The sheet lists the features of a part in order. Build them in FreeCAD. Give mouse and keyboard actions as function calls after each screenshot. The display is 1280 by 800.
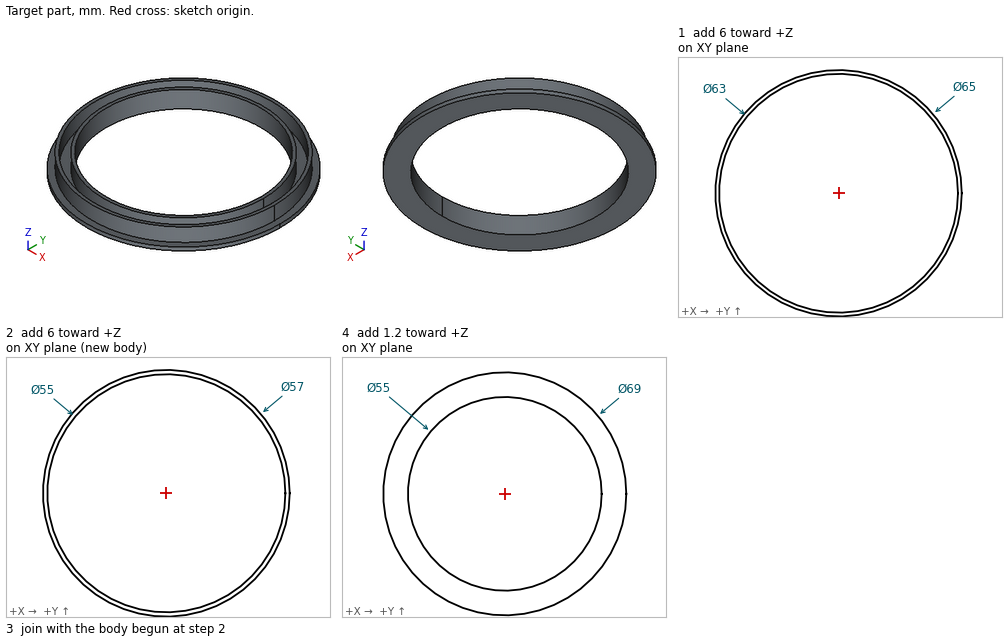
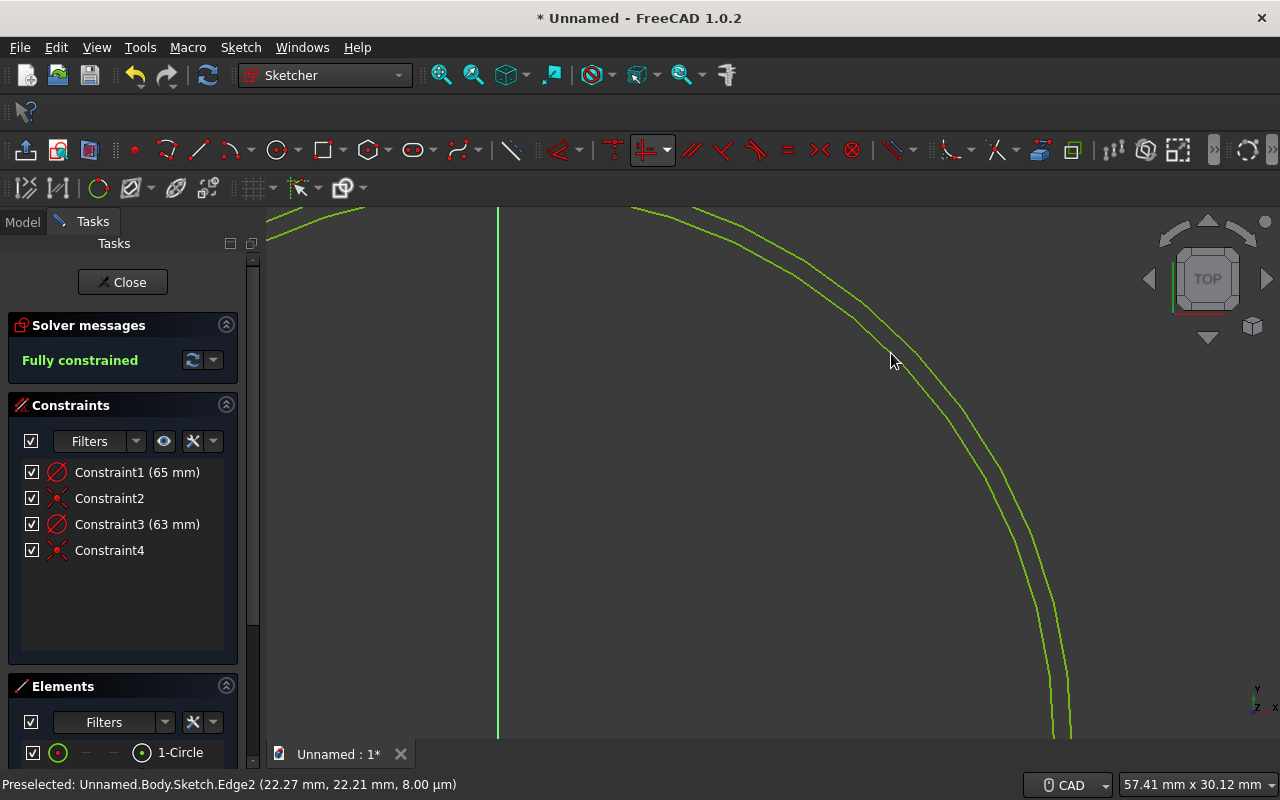
click(123, 282)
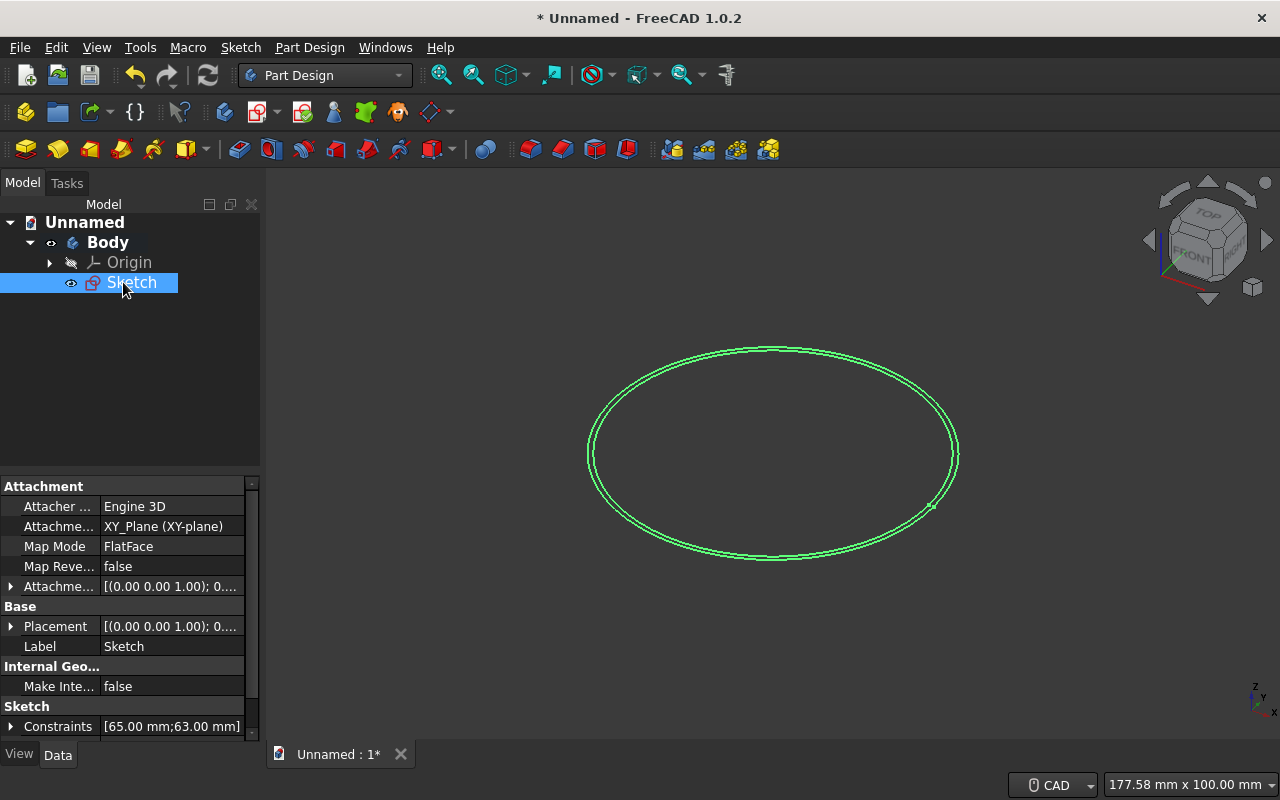
click(26, 150)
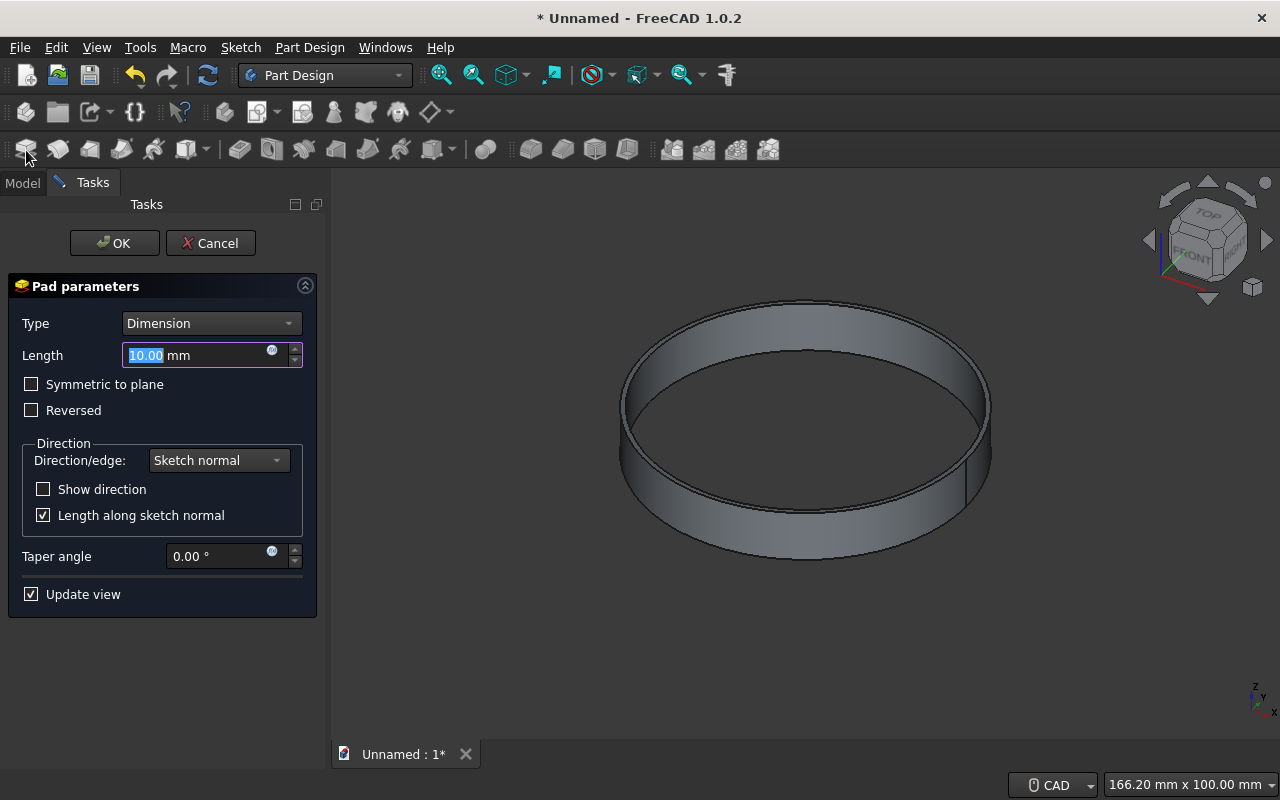
text(6)
key(Tab)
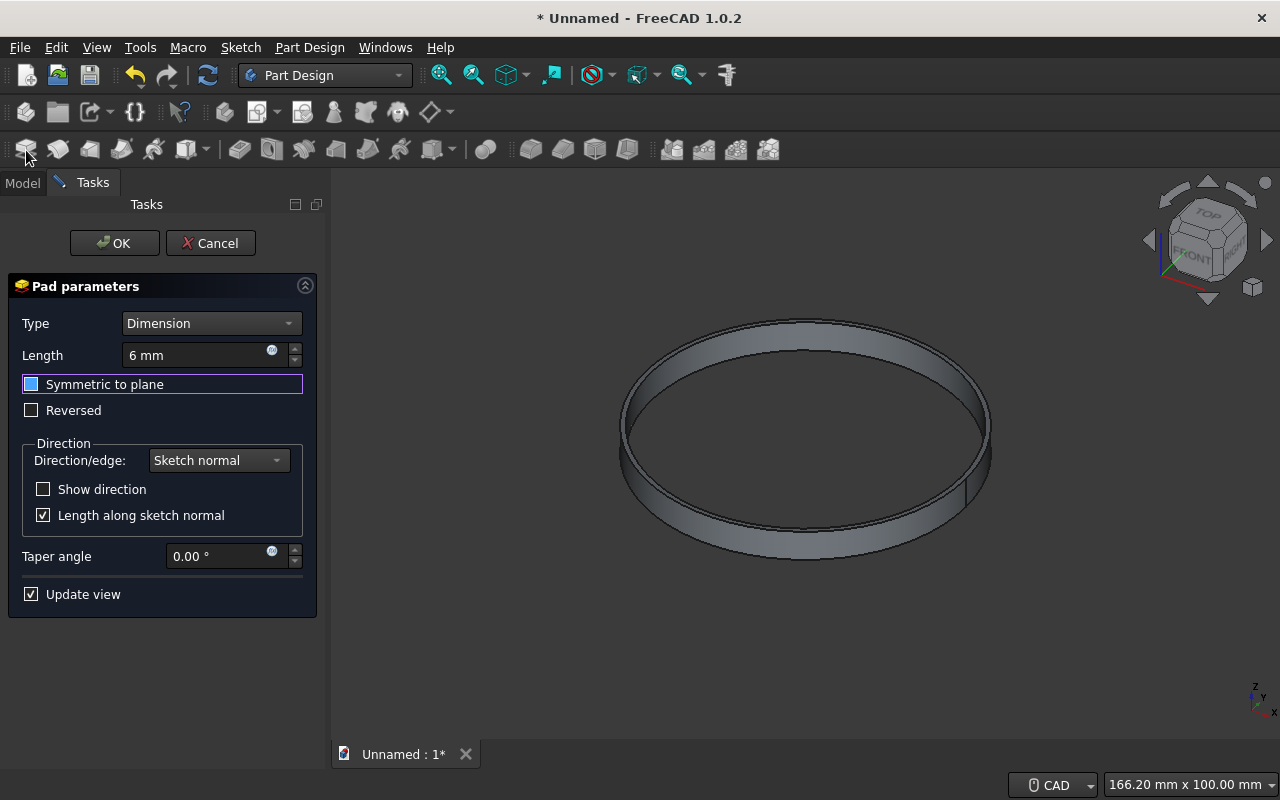
click(115, 243)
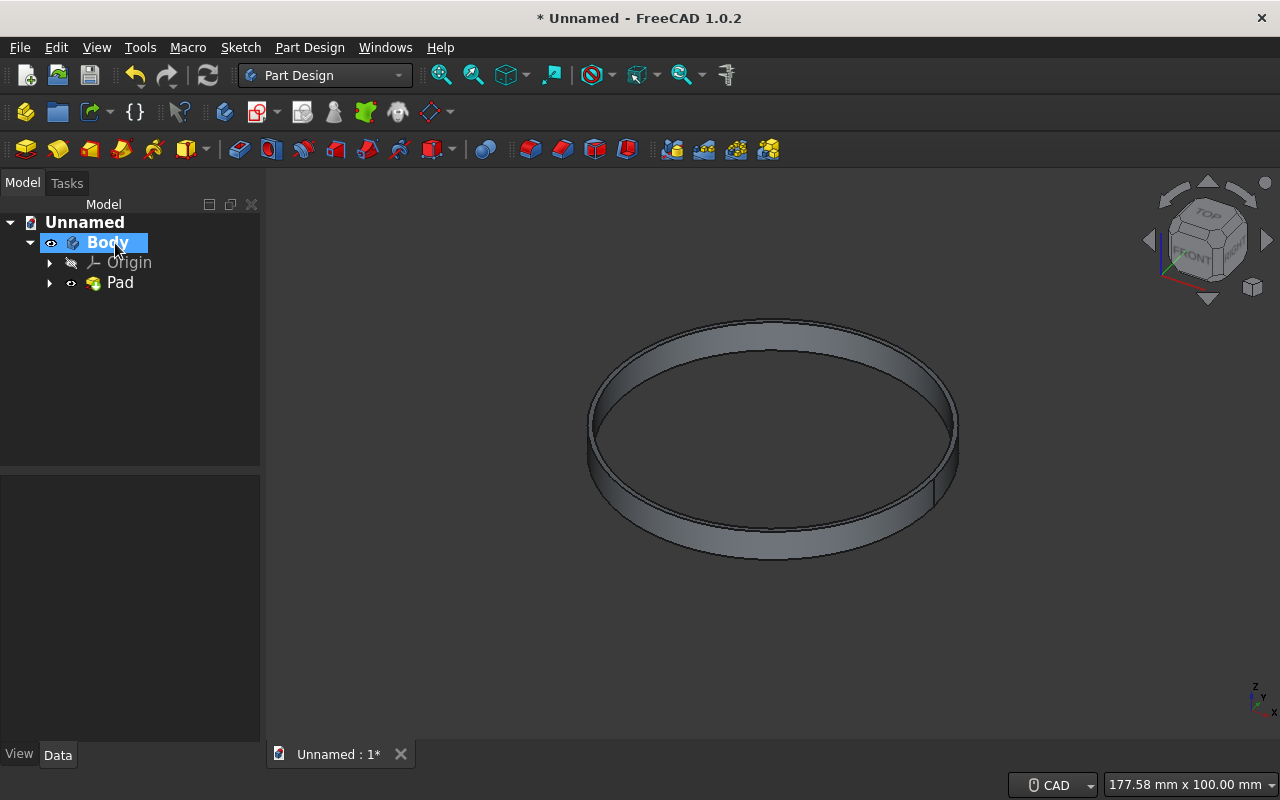
click(226, 112)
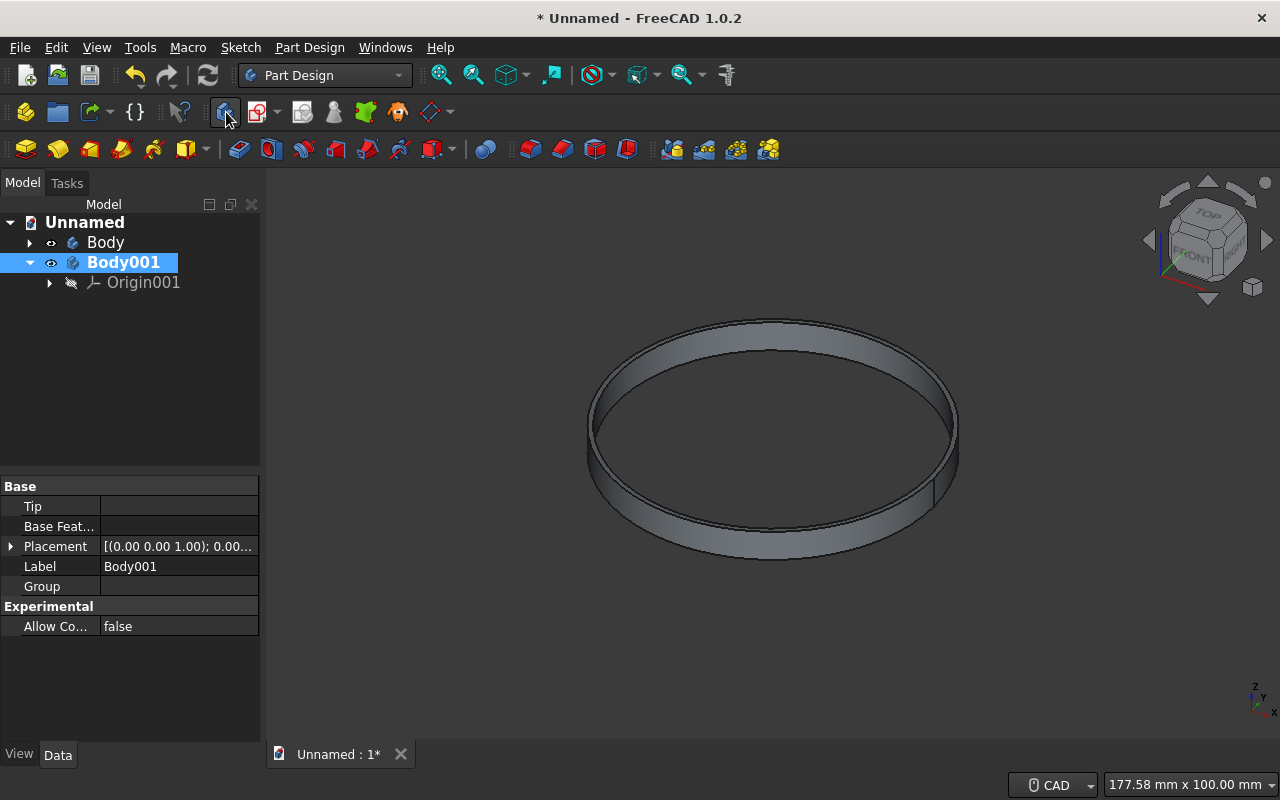
click(306, 699)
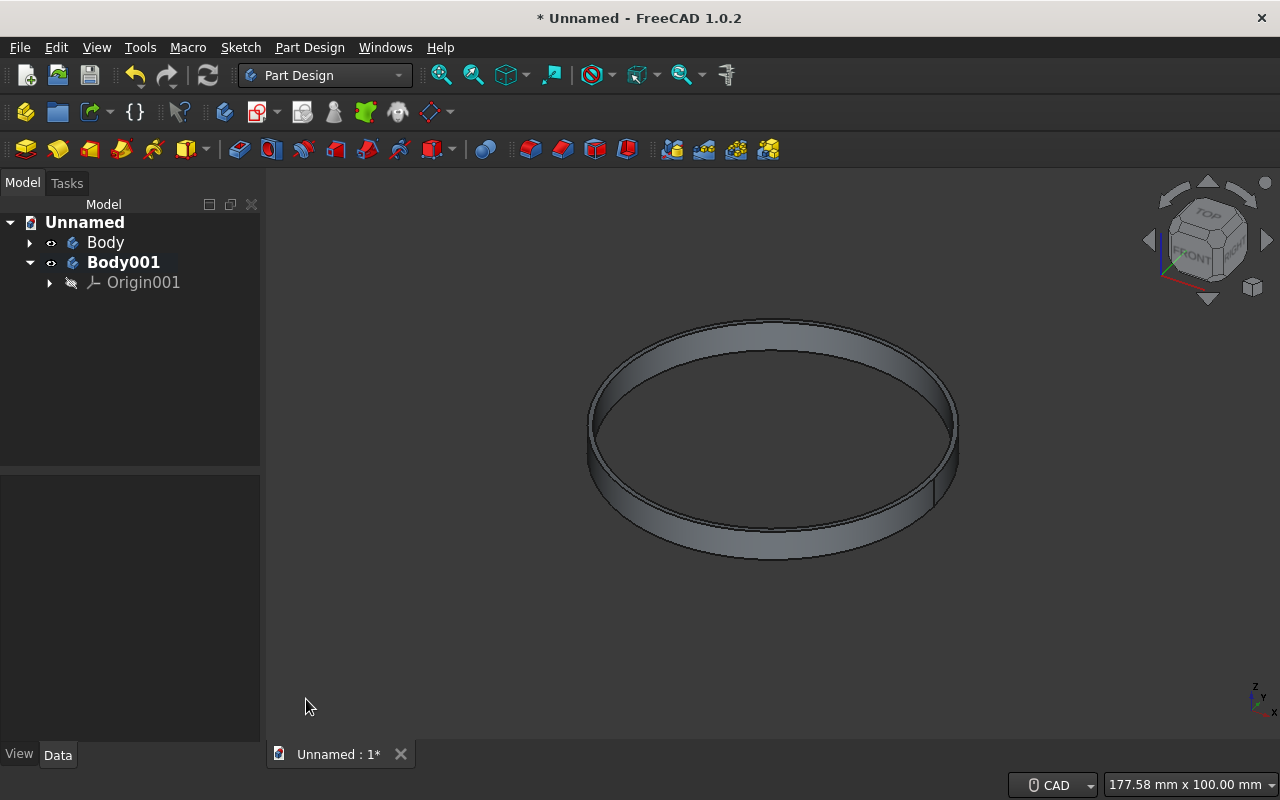
click(258, 112)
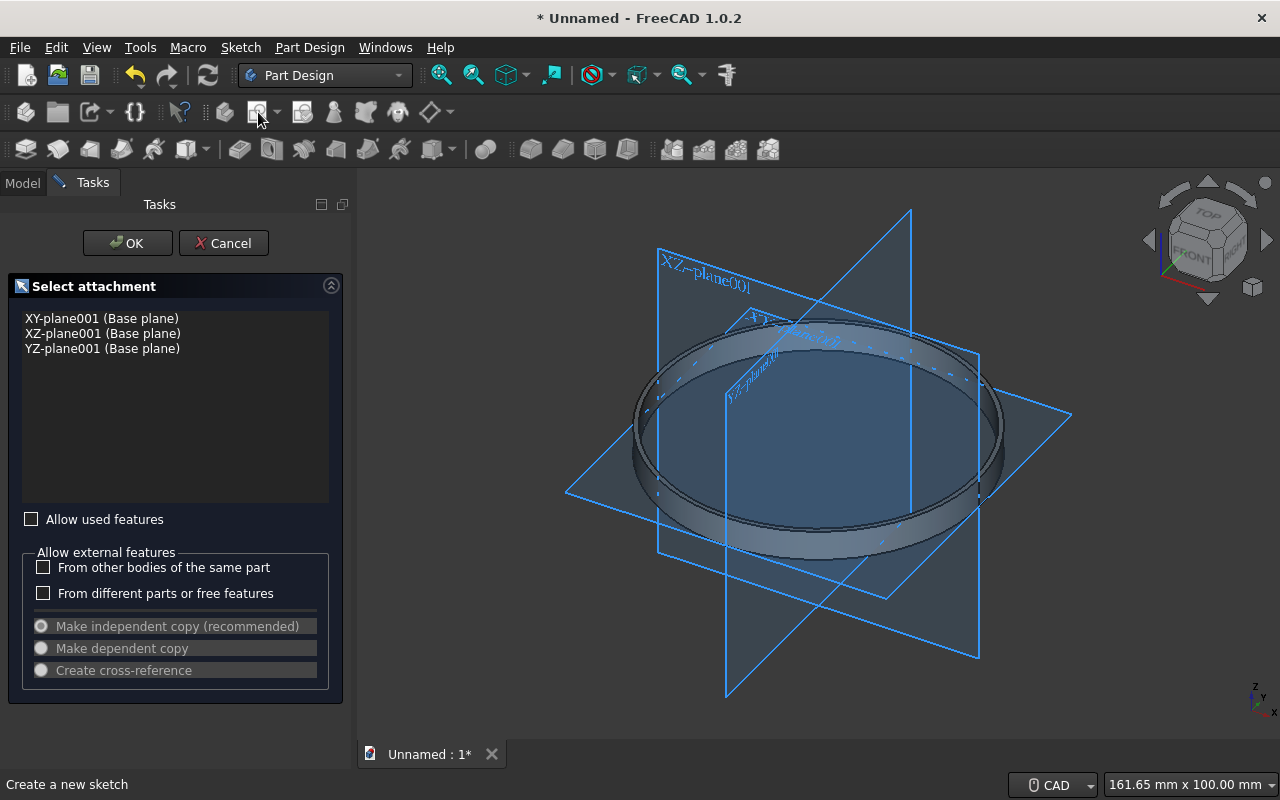
click(82, 318)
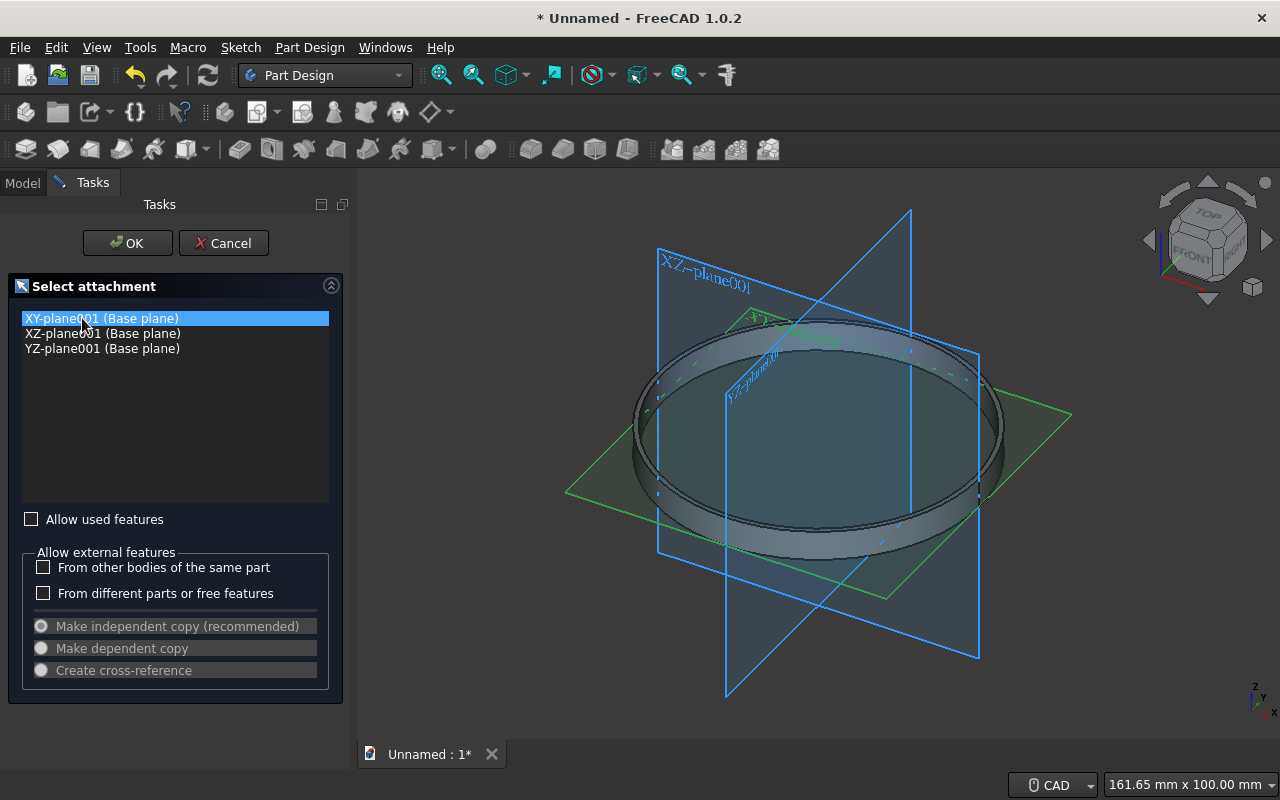
click(128, 243)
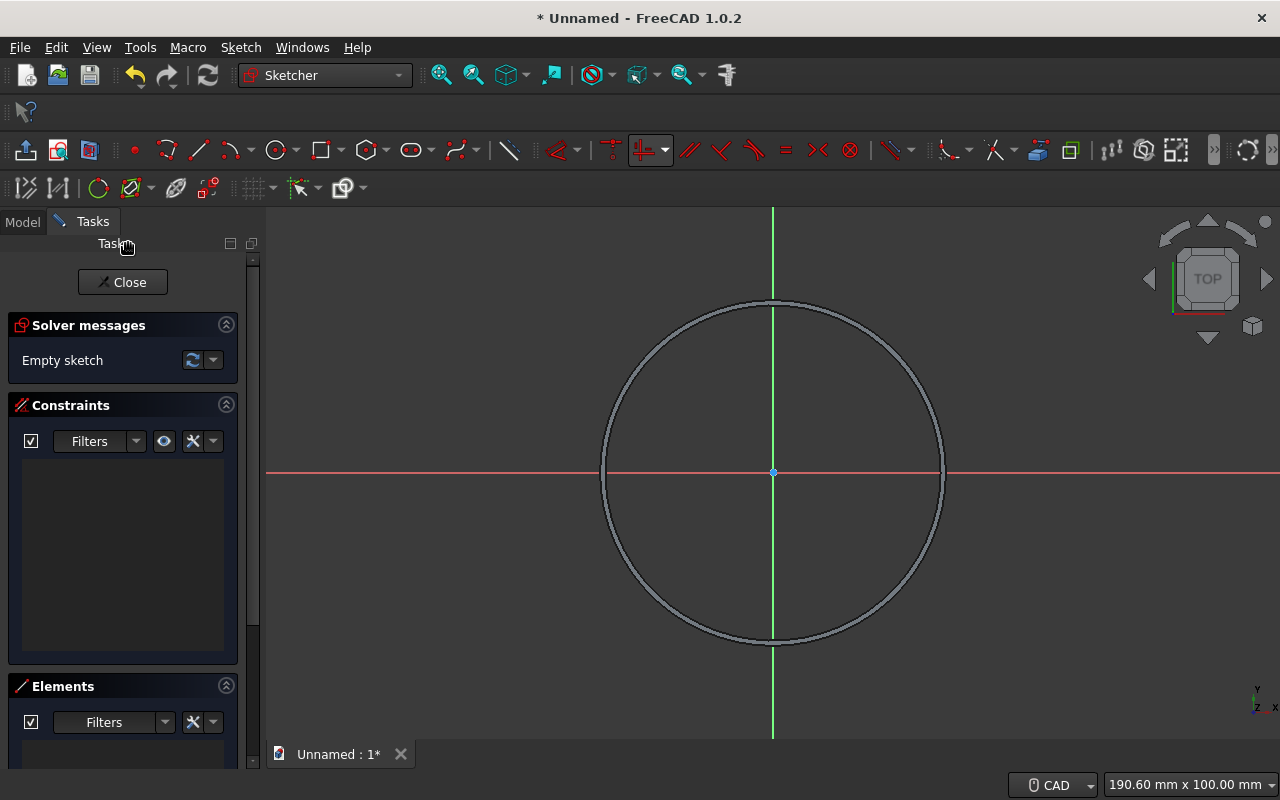
click(276, 150)